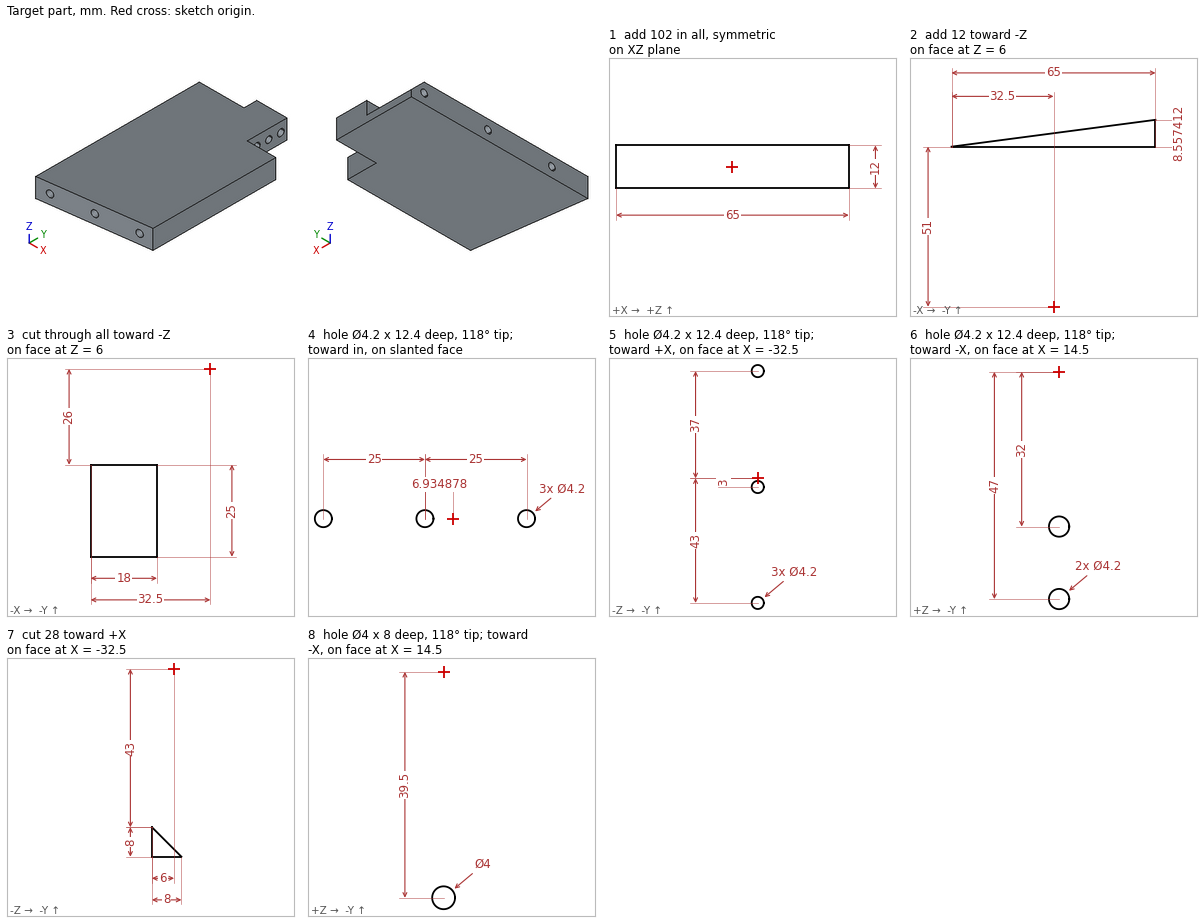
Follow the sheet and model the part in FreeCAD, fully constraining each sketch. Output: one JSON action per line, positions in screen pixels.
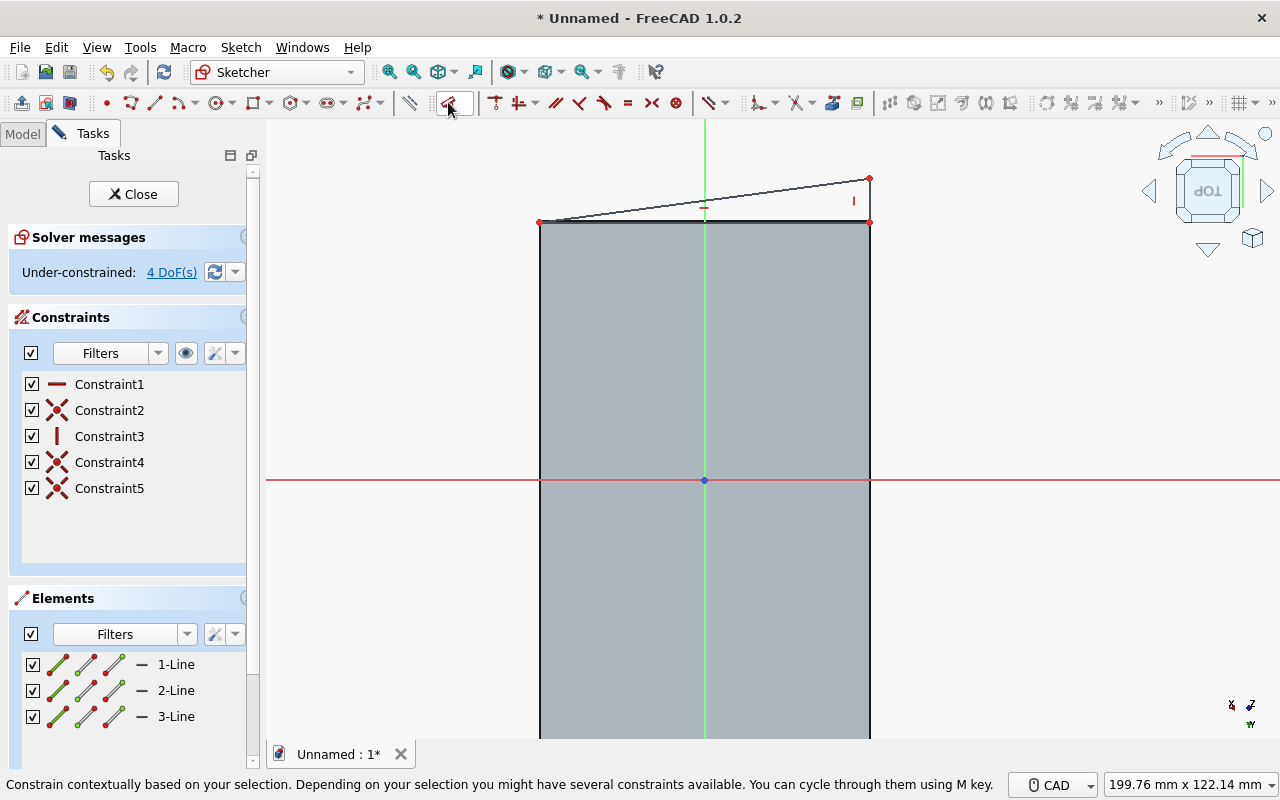
{"action": "left_click", "coordinate": [639, 223]}
{"action": "left_click", "coordinate": [629, 189]}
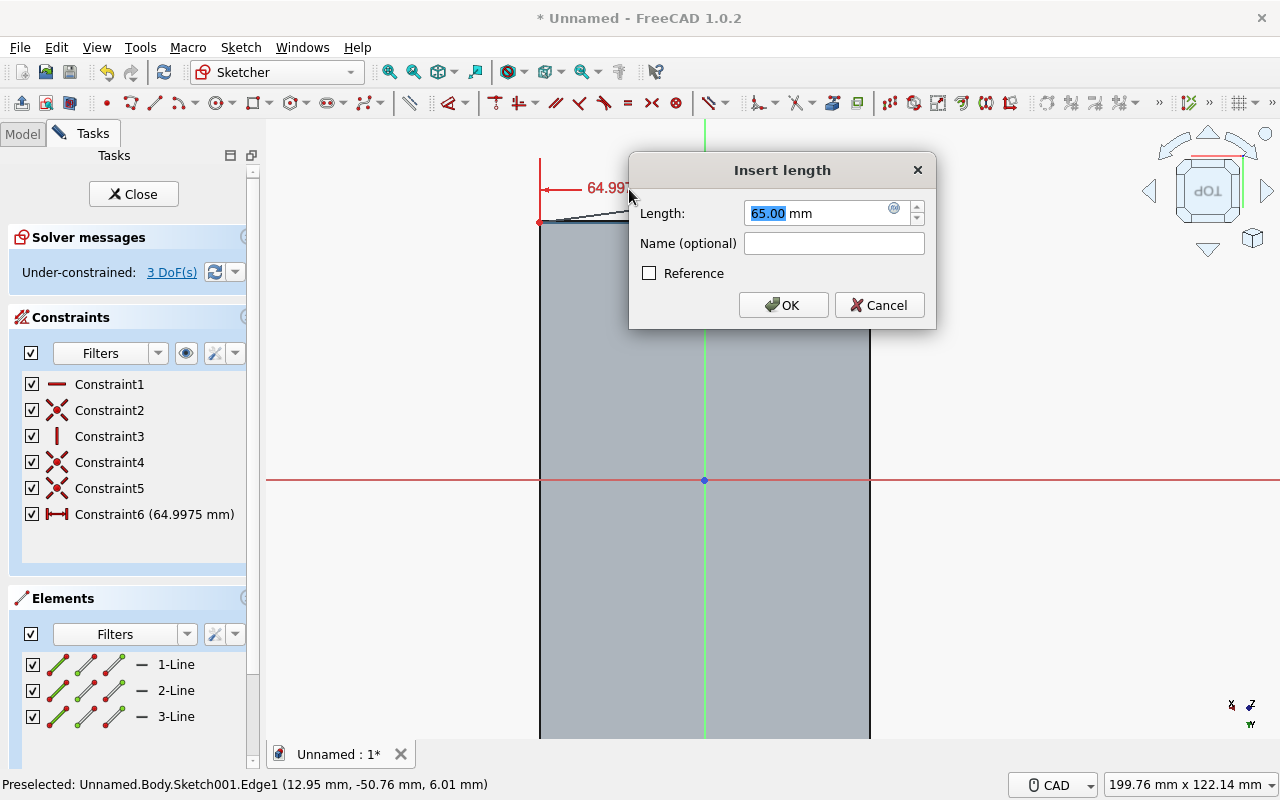
{"action": "type", "text": "65"}
{"action": "key", "text": "Return"}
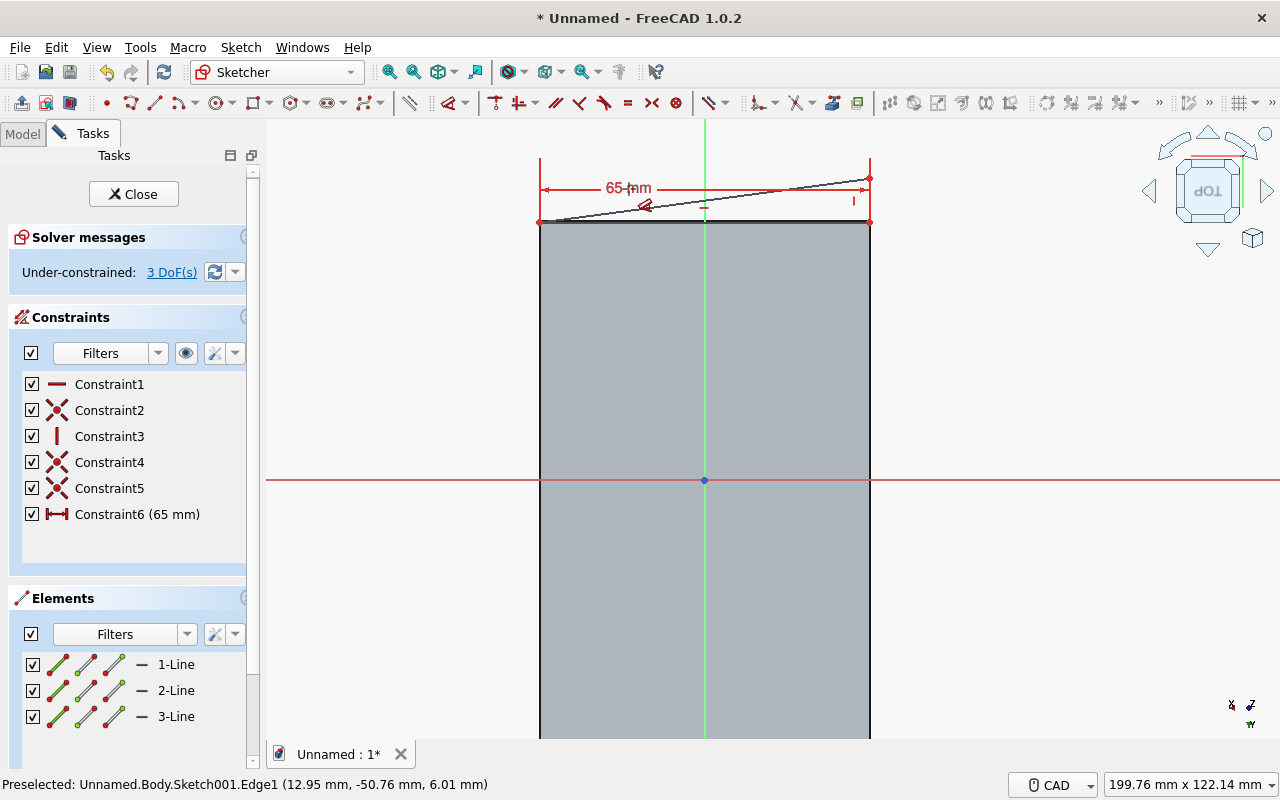
{"action": "left_click", "coordinate": [540, 223]}
{"action": "left_click", "coordinate": [506, 351]}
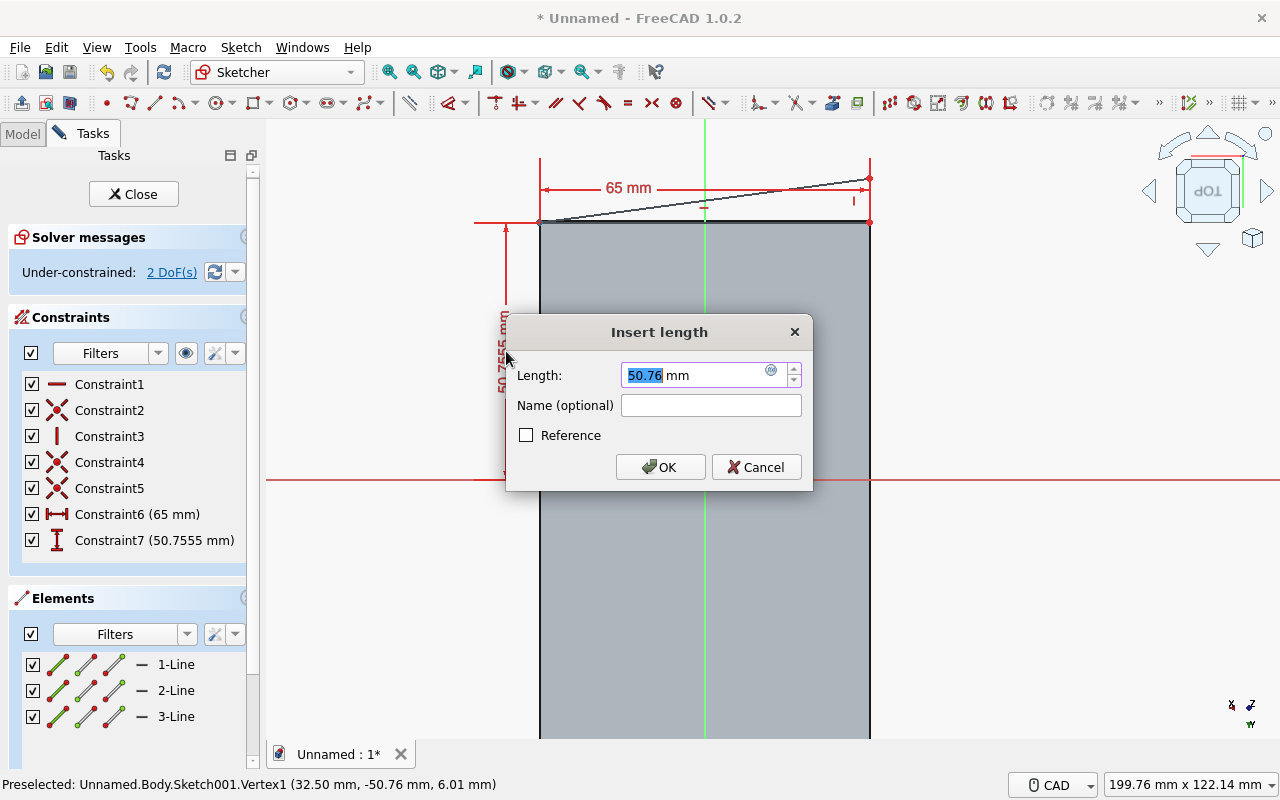
{"action": "type", "text": "51"}
{"action": "key", "text": "Return"}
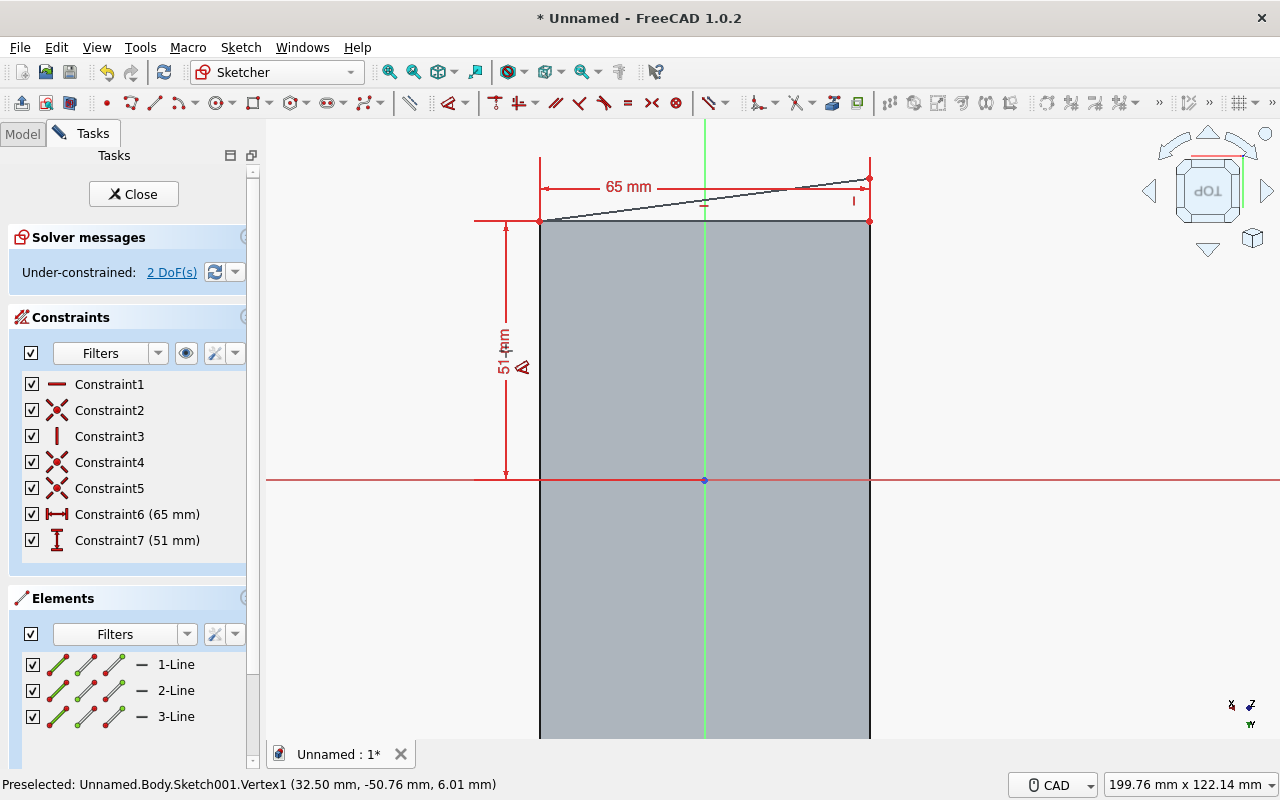
{"action": "left_click", "coordinate": [540, 221]}
{"action": "left_click", "coordinate": [622, 514]}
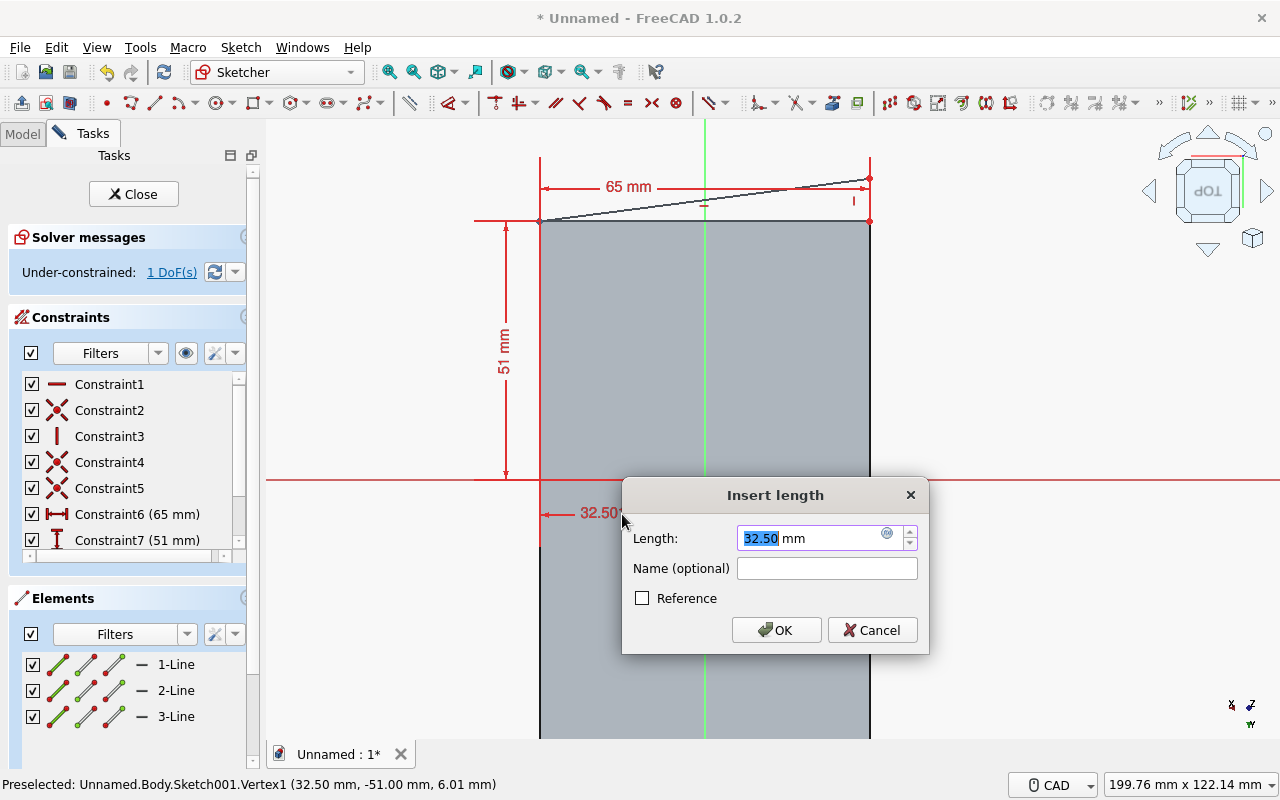
{"action": "type", "text": "32.5"}
{"action": "key", "text": "Return"}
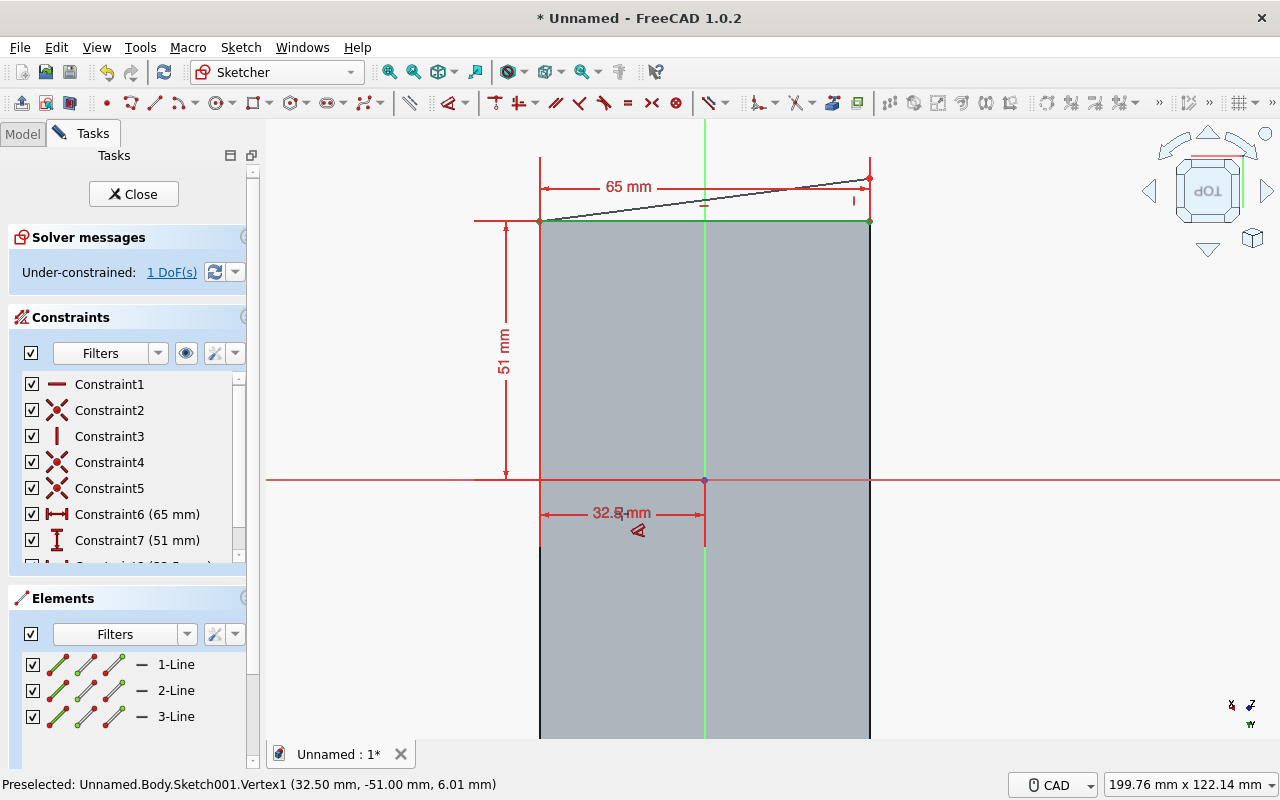
{"action": "left_click", "coordinate": [870, 209]}
{"action": "left_click", "coordinate": [904, 200]}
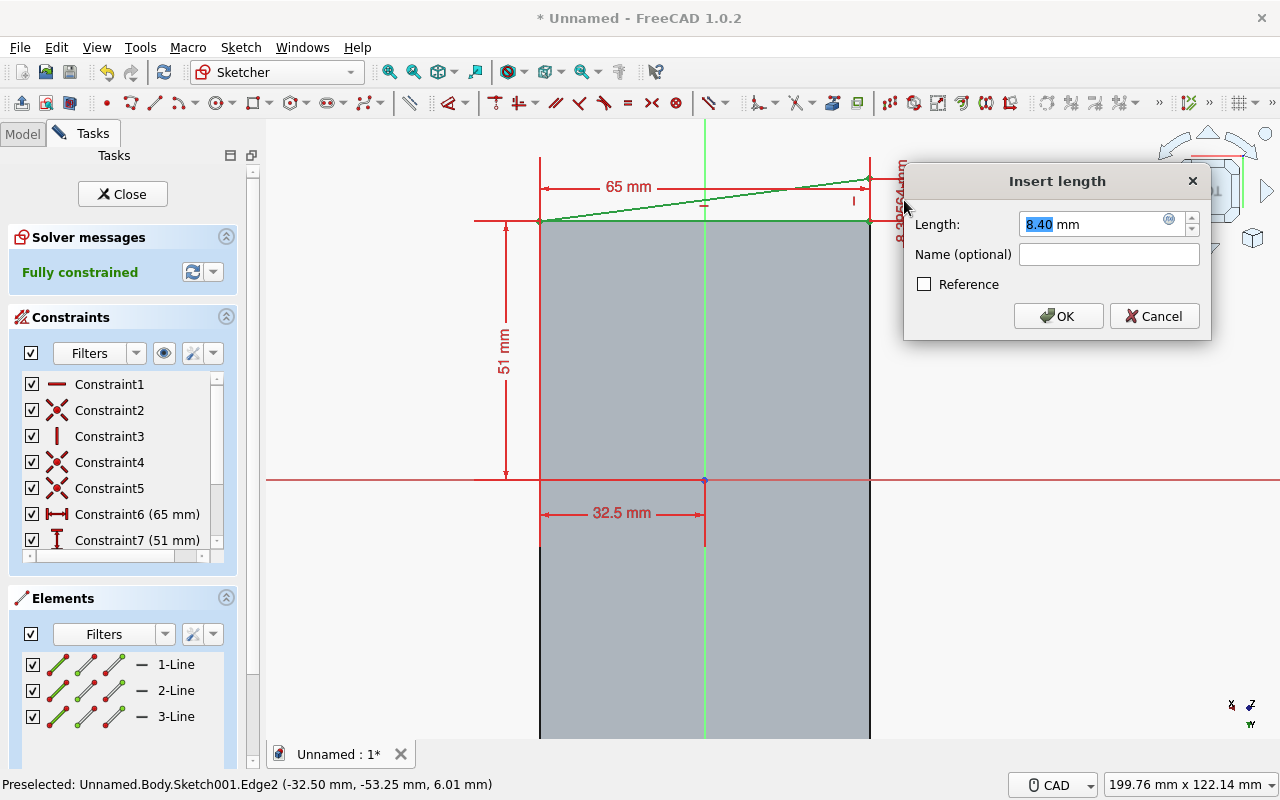
{"action": "type", "text": "8.557412"}
{"action": "key", "text": "Return"}
{"action": "key", "text": "Escape"}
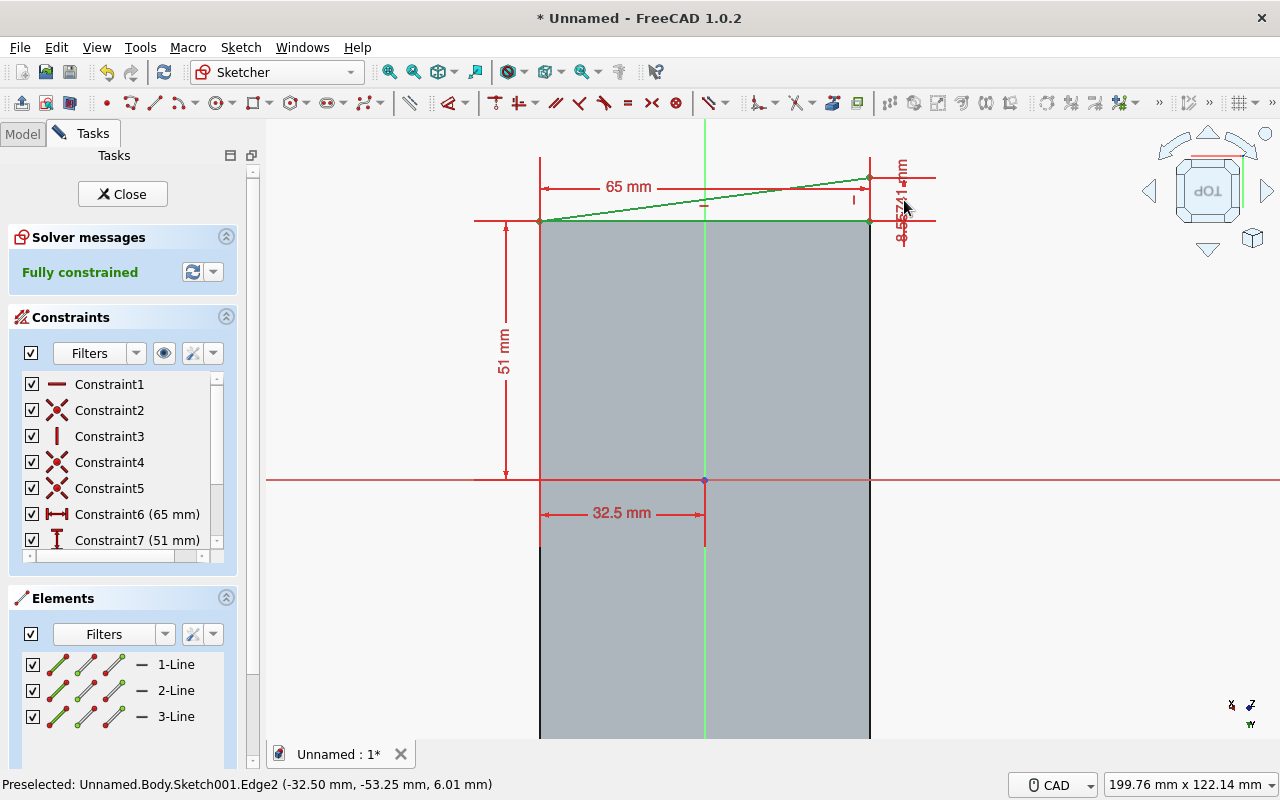
{"action": "left_click", "coordinate": [123, 194]}